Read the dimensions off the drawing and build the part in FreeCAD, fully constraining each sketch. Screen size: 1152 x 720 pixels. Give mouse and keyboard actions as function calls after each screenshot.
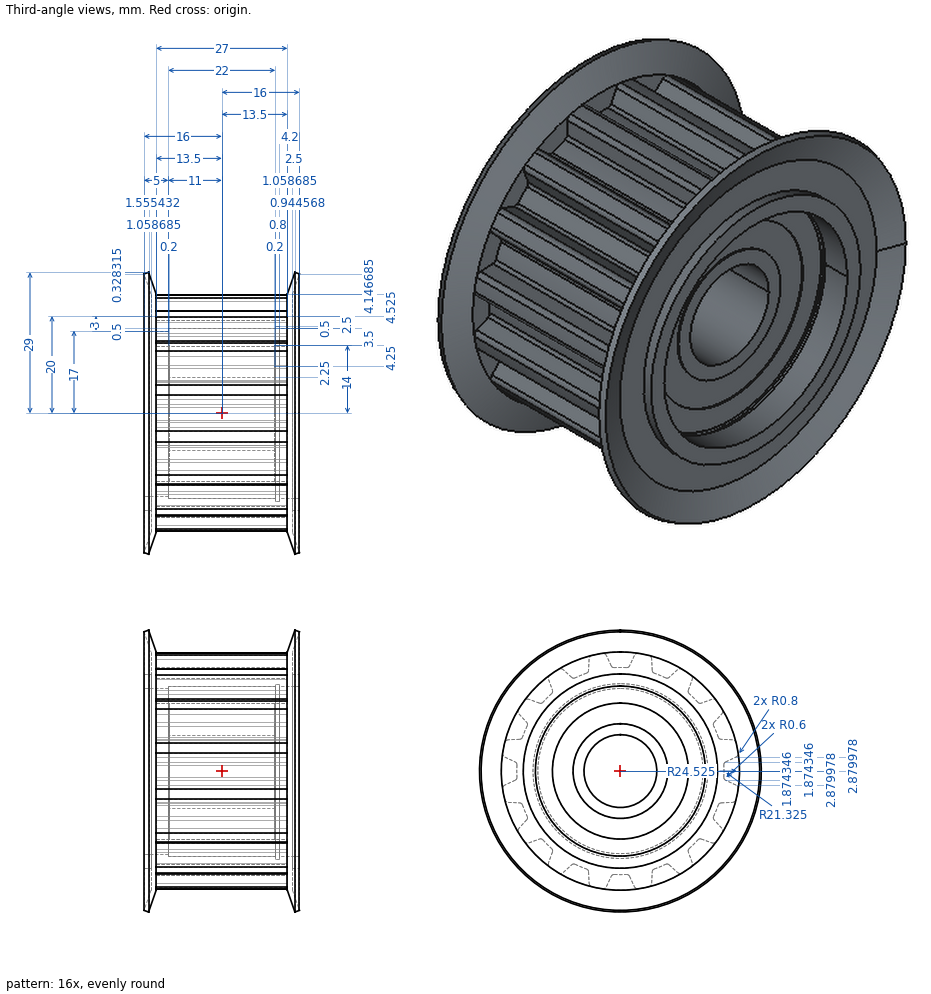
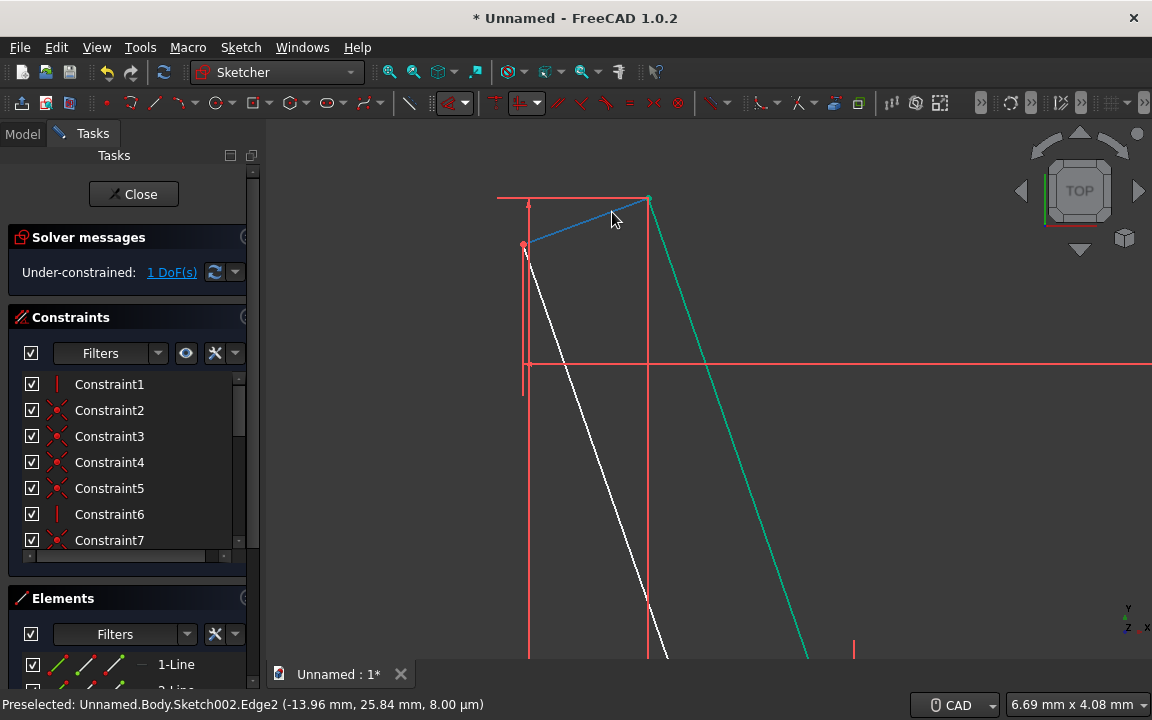
click(611, 212)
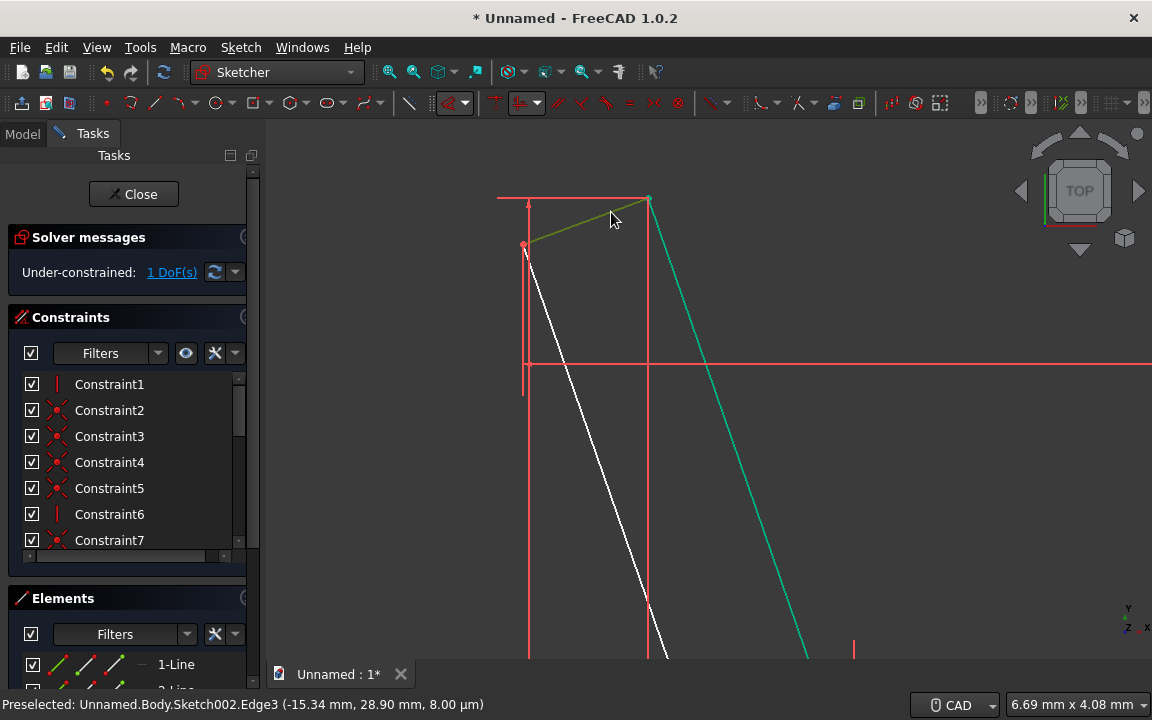
click(468, 104)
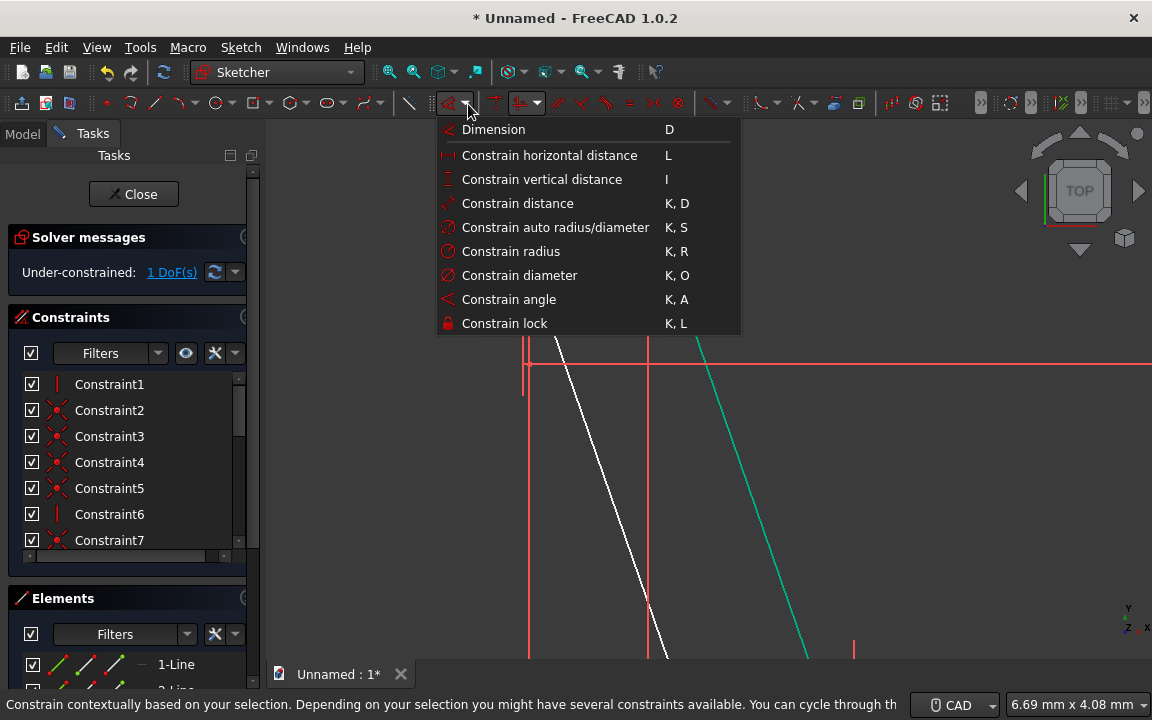
click(589, 179)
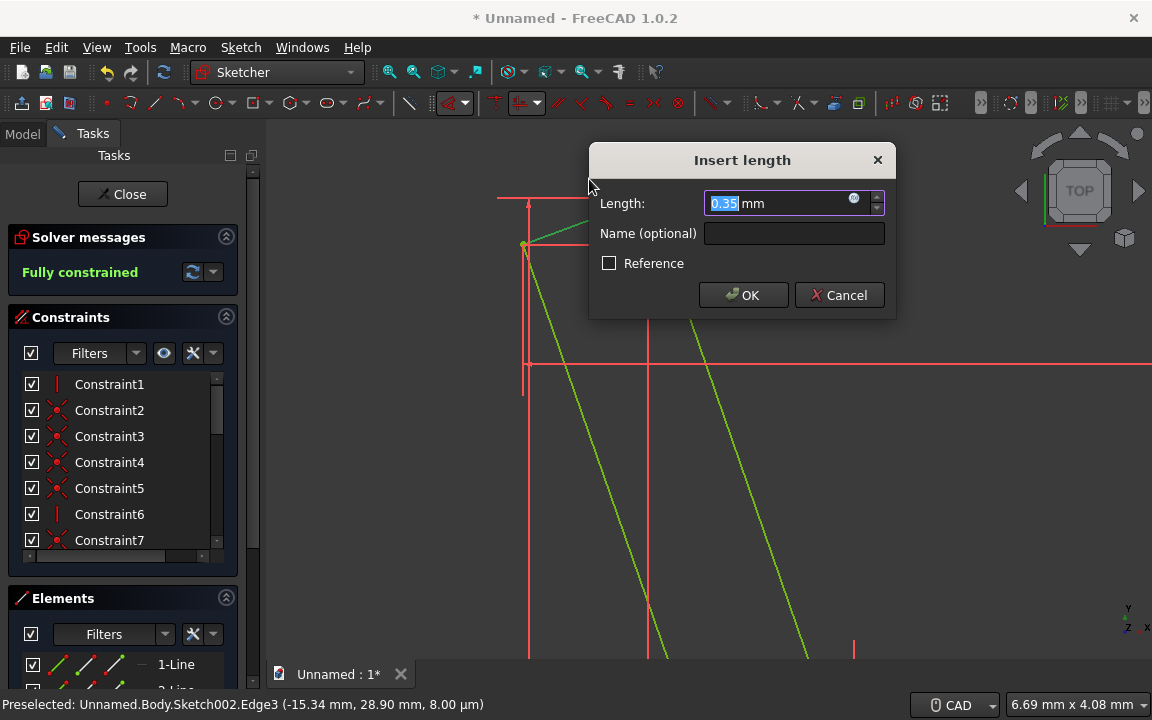
text(0.328315)
key(Return)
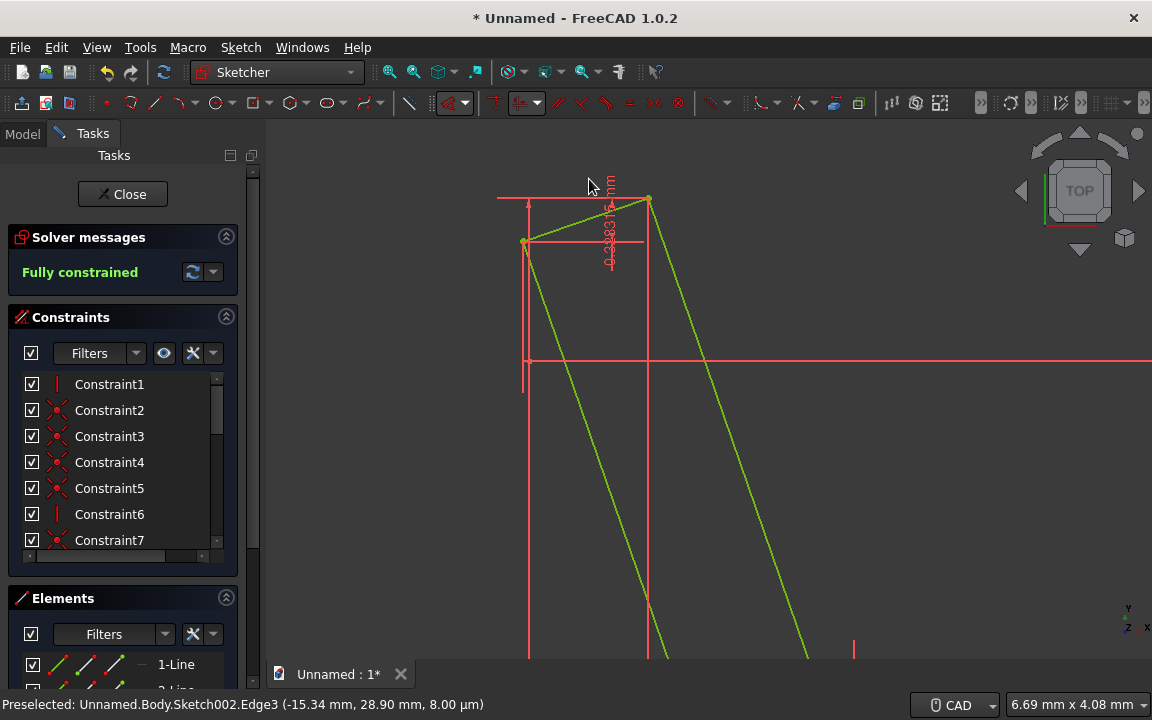
click(123, 194)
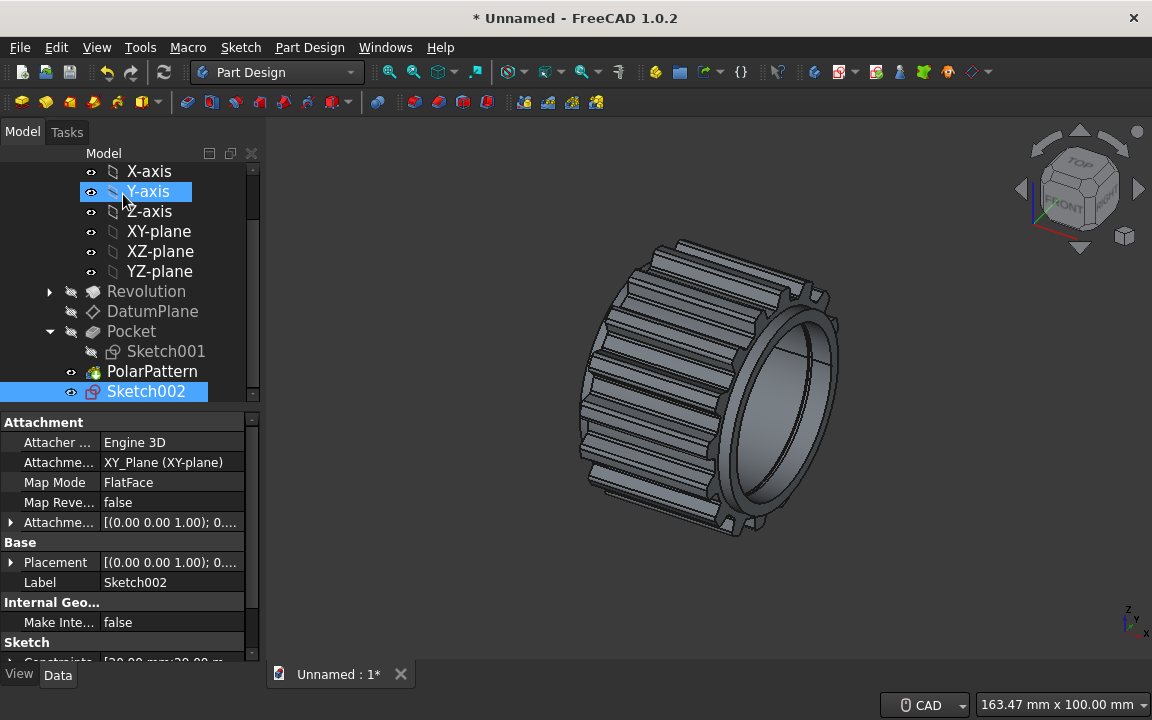
click(46, 102)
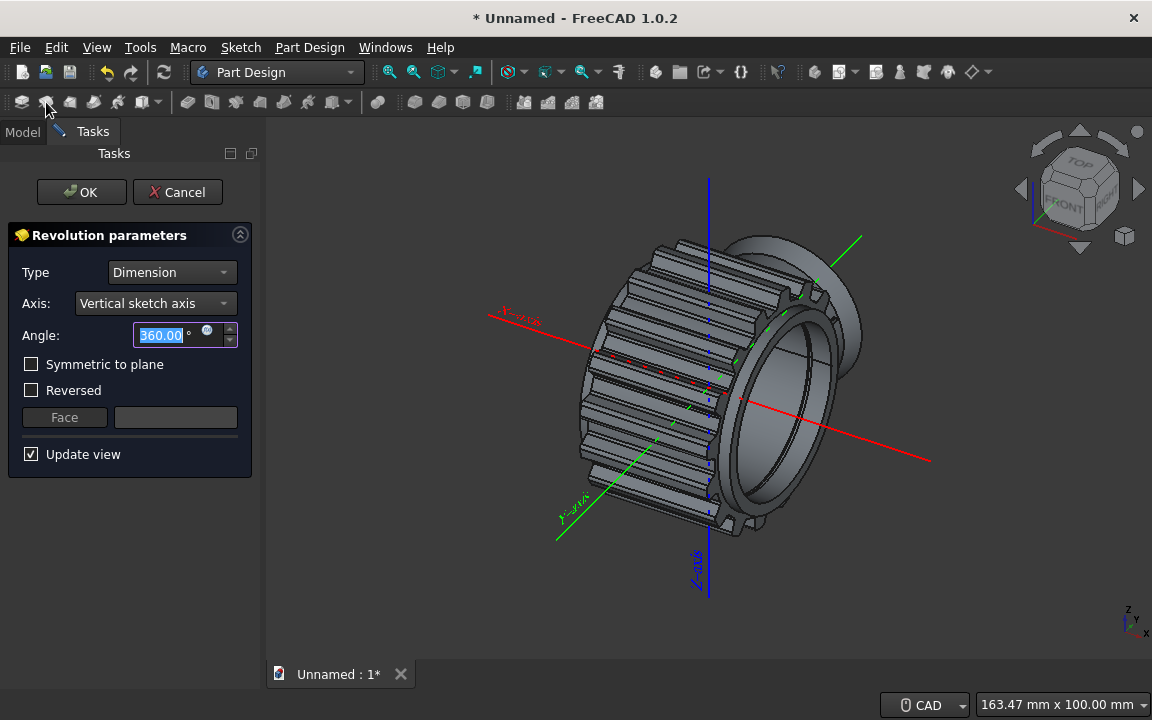
click(156, 304)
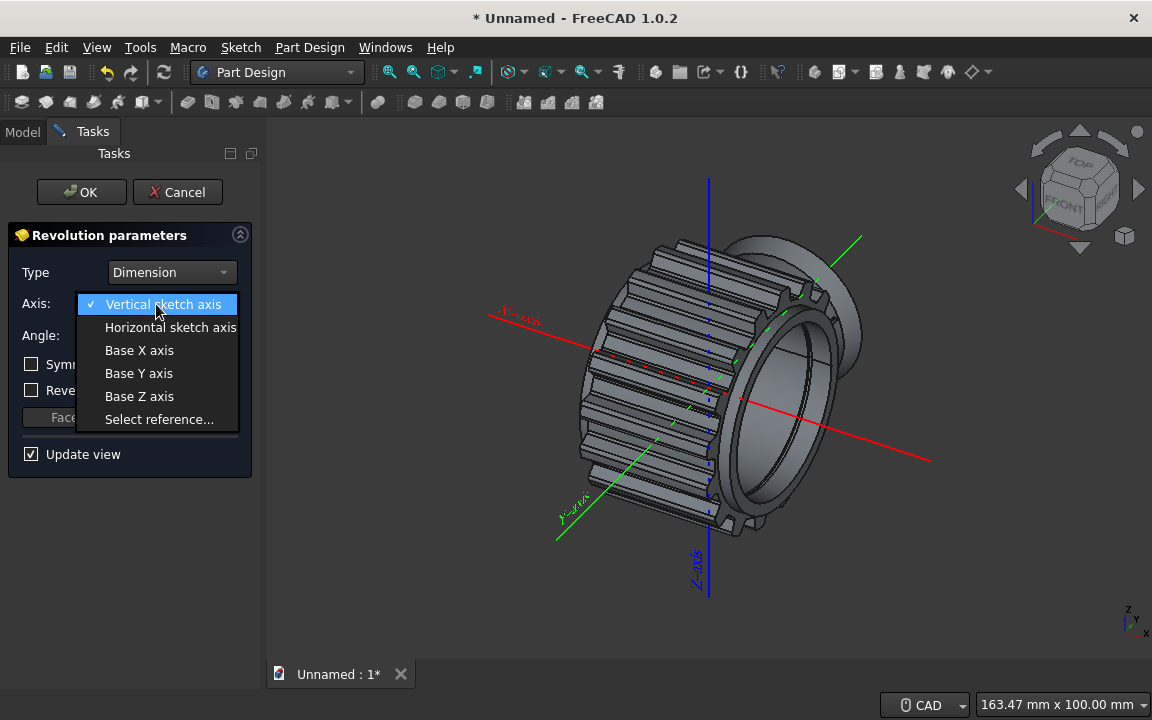
click(156, 328)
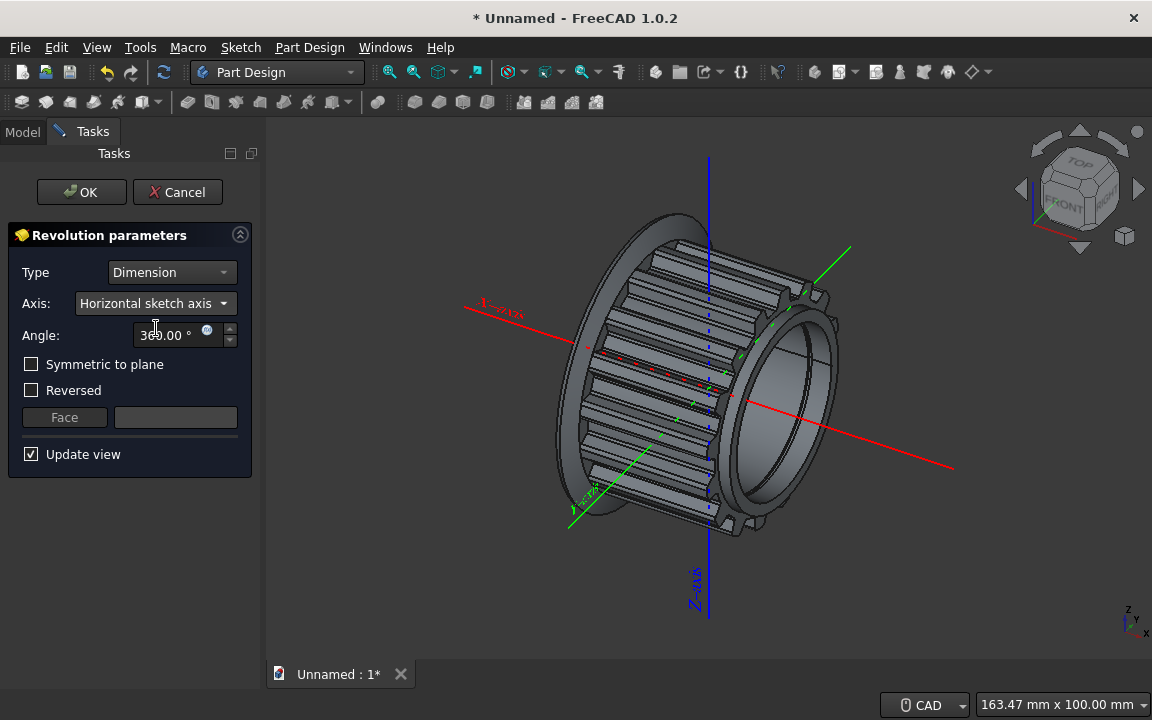
click(82, 192)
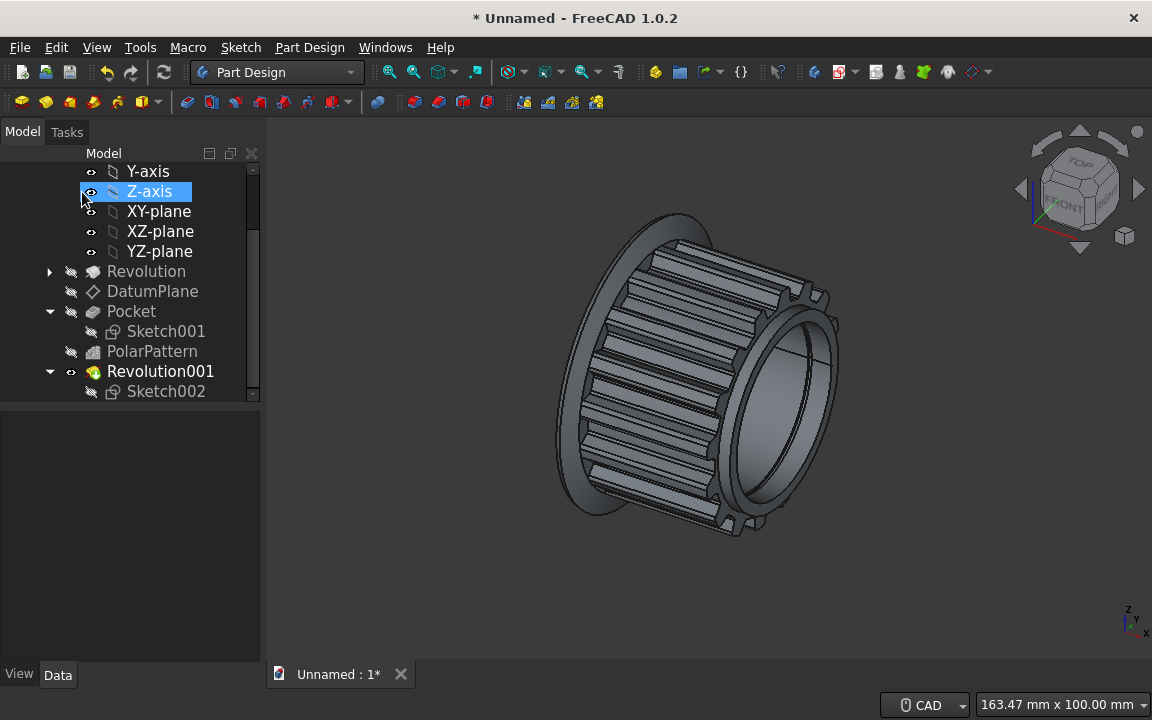
click(840, 72)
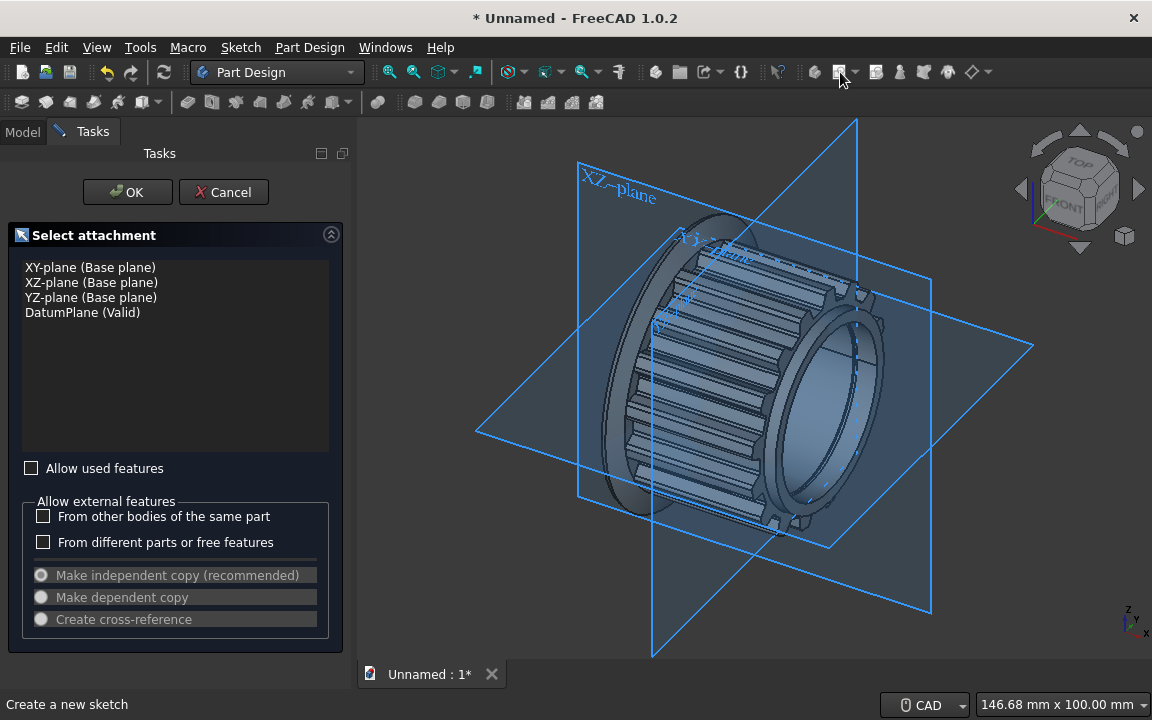
click(82, 268)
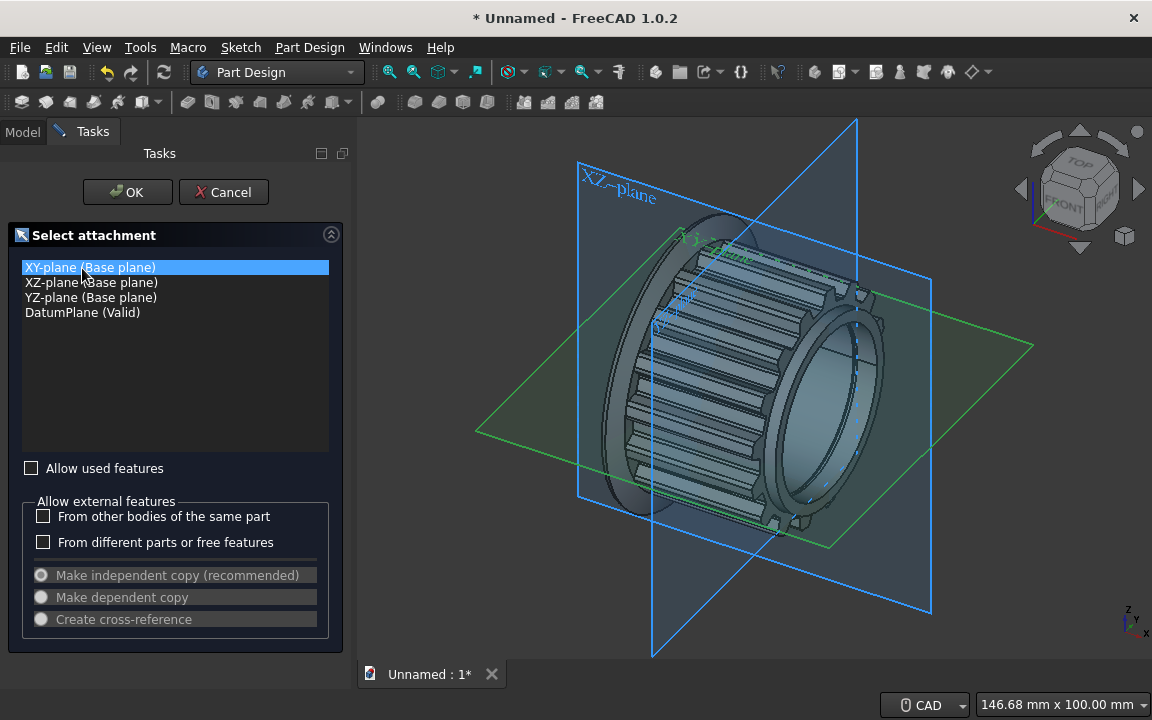
click(128, 192)